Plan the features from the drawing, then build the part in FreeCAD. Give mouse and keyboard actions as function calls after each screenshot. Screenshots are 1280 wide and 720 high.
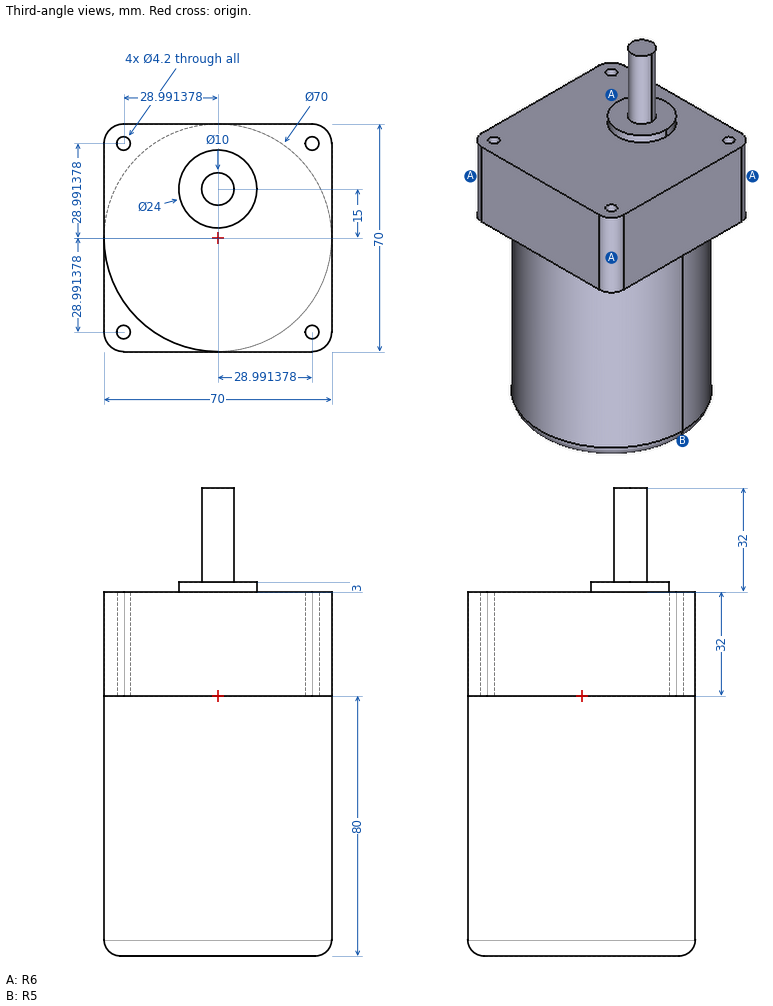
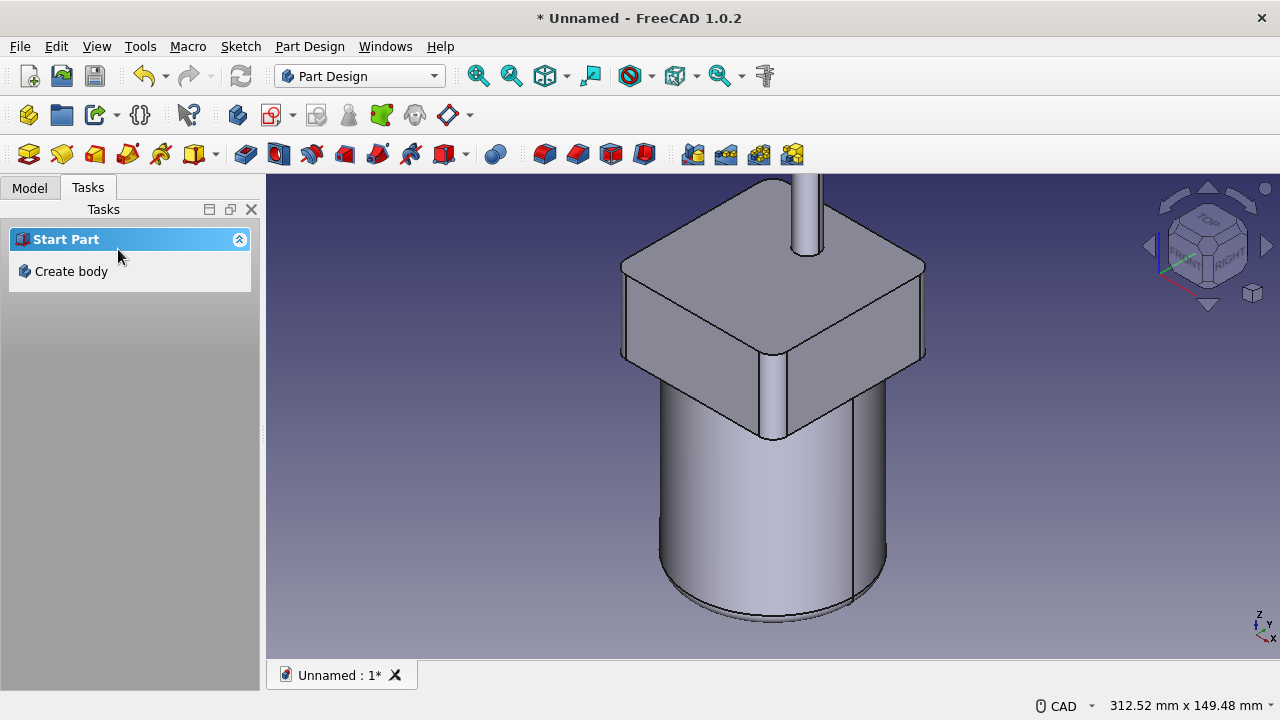
click(479, 76)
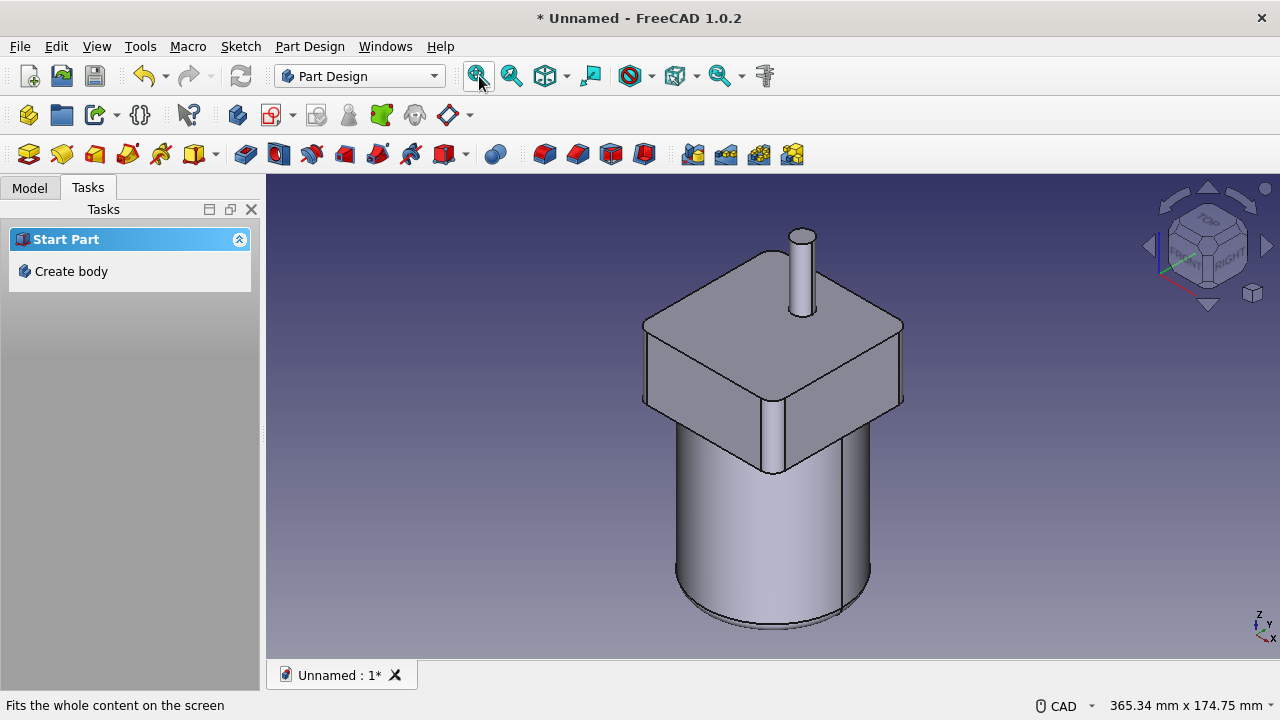
click(773, 348)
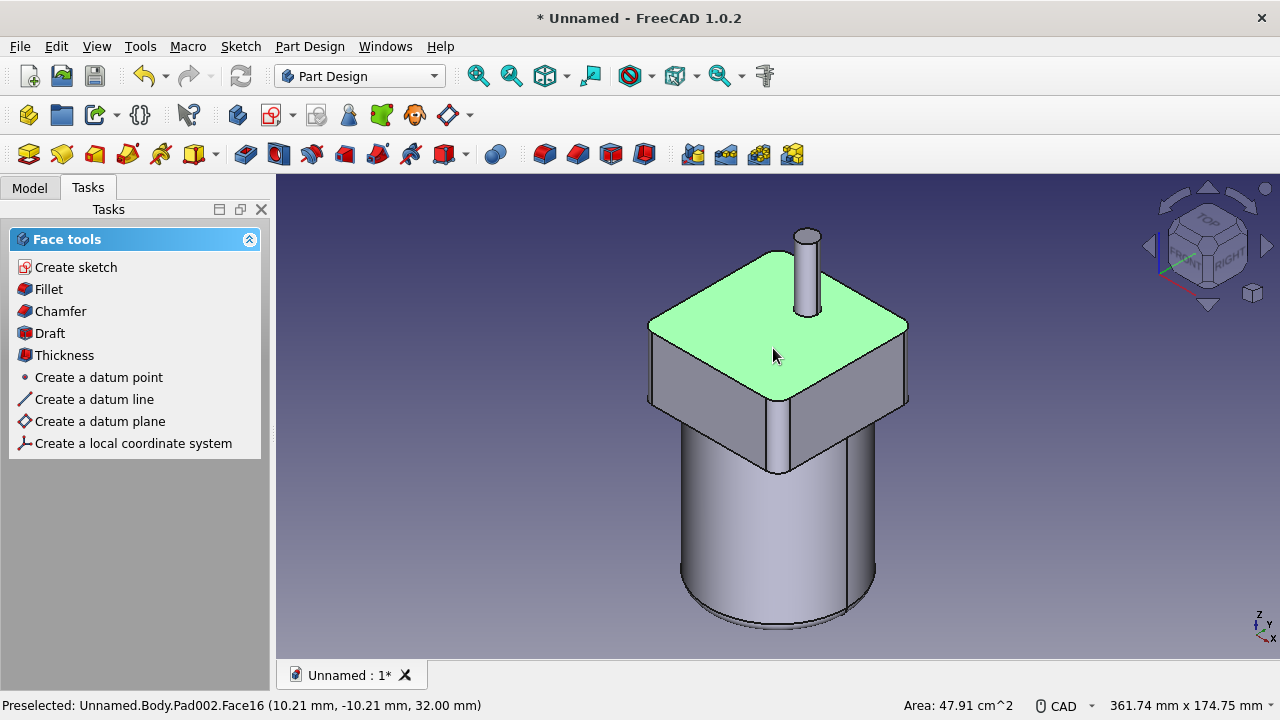
click(270, 116)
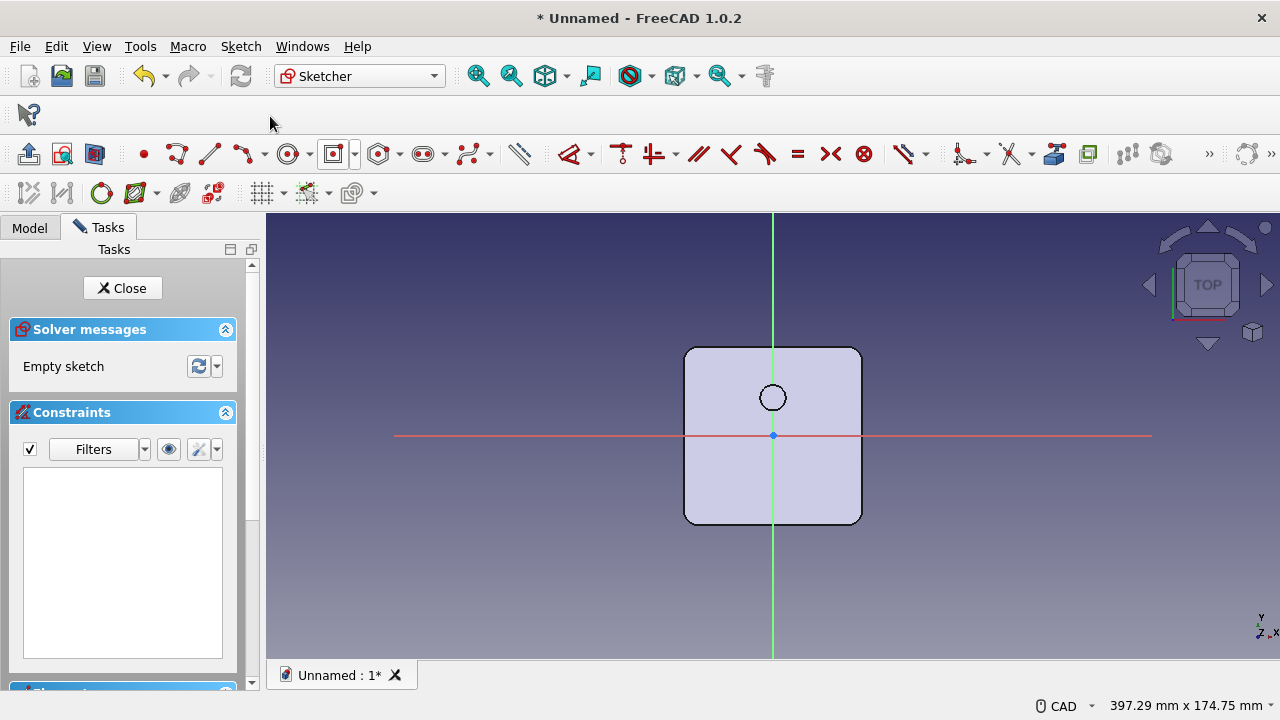
click(95, 154)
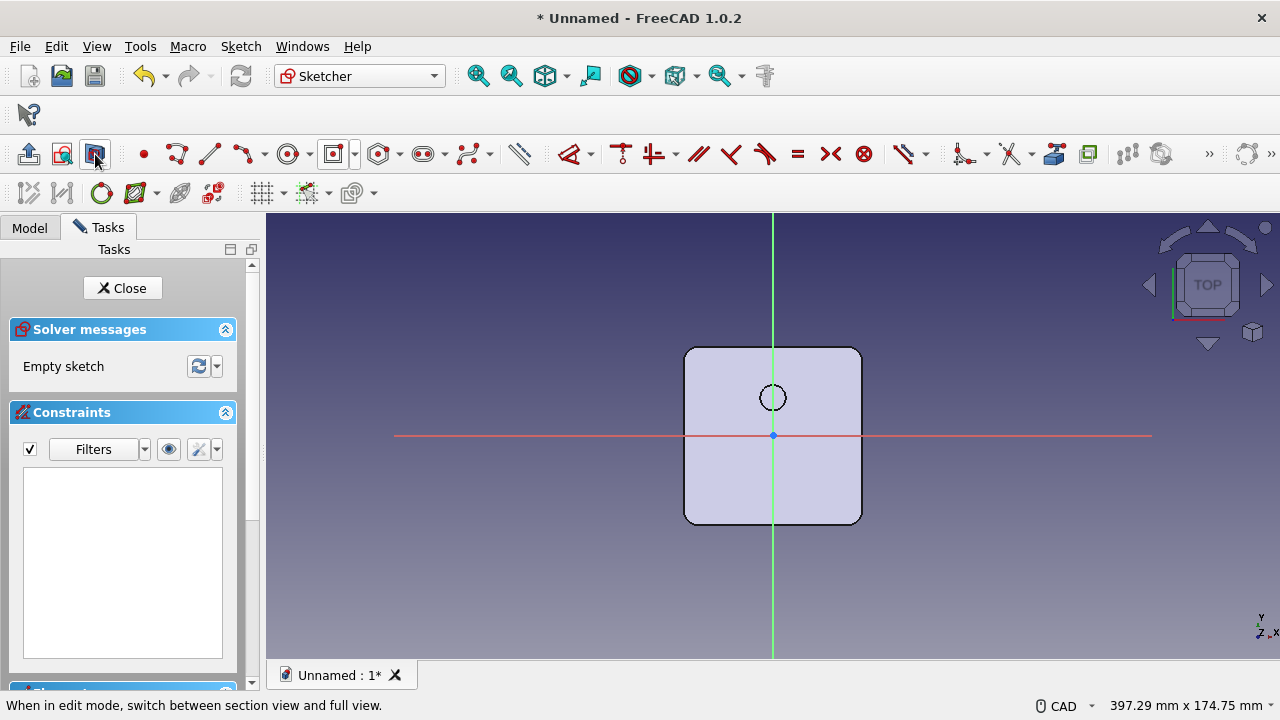
scroll(856, 436, up, 3)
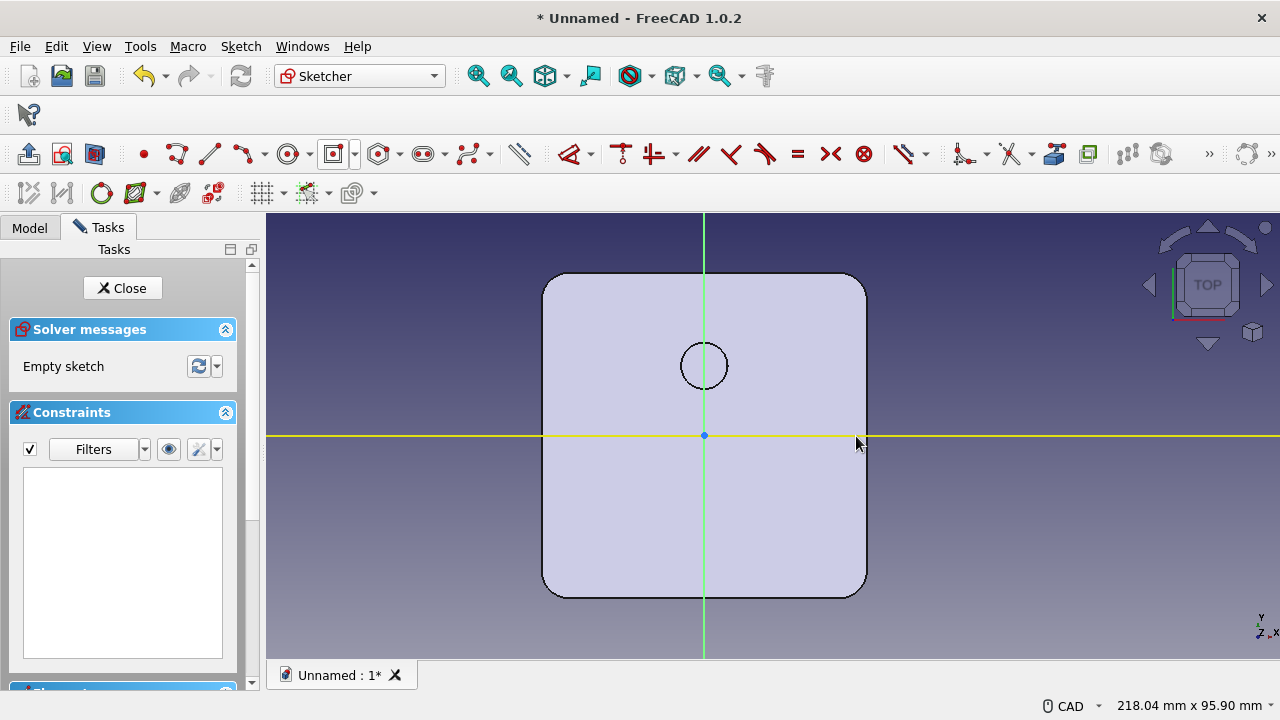
click(288, 154)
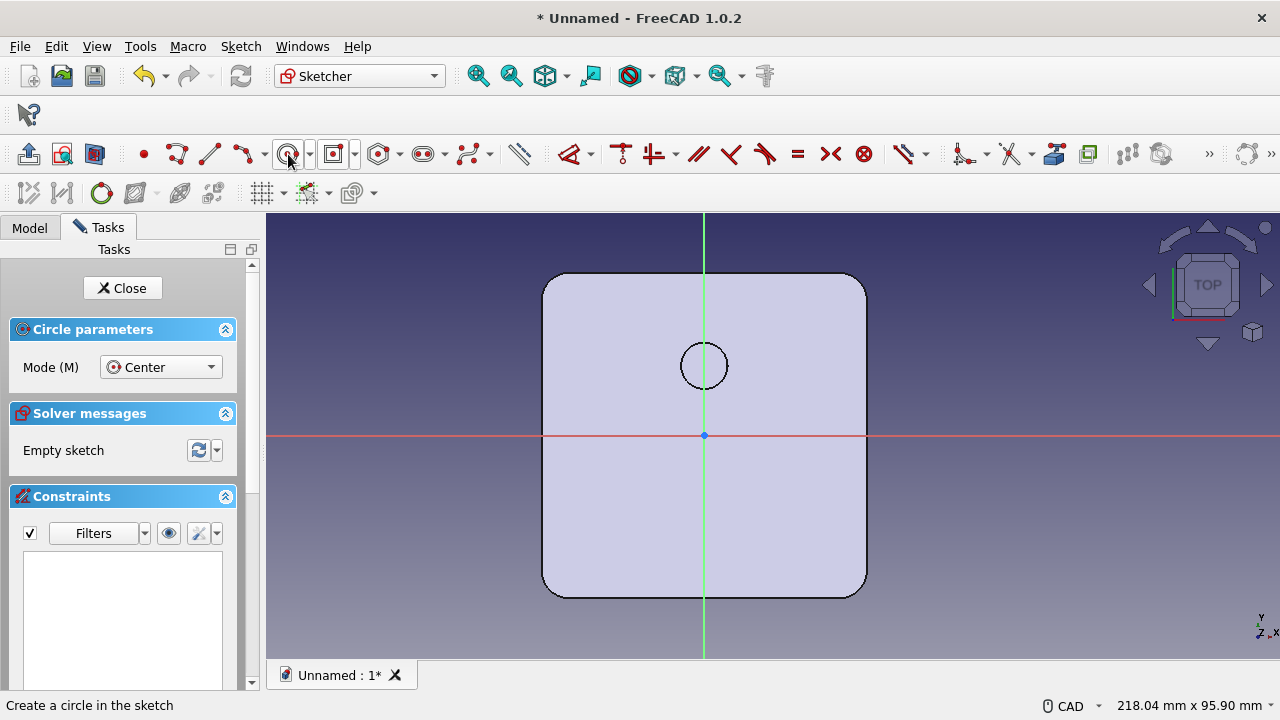
scroll(569, 301, up, 5)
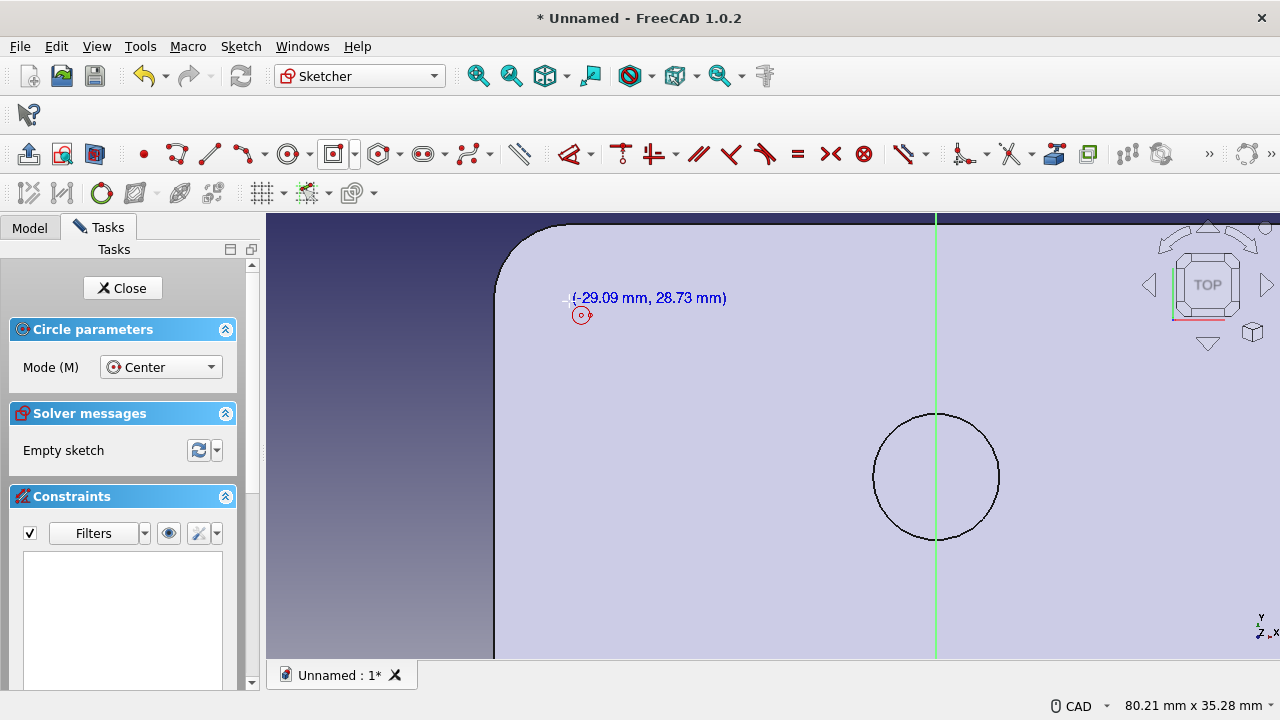
click(570, 300)
move(589, 281)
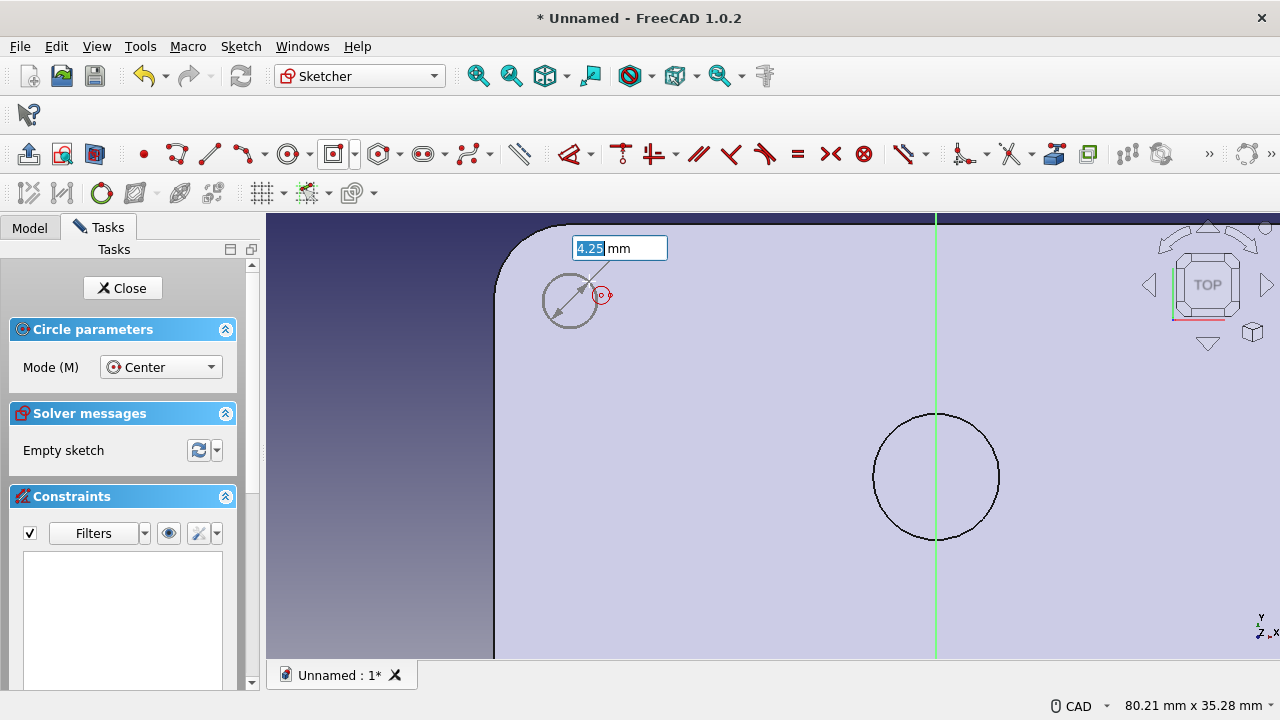
text(4.2)
key(Return)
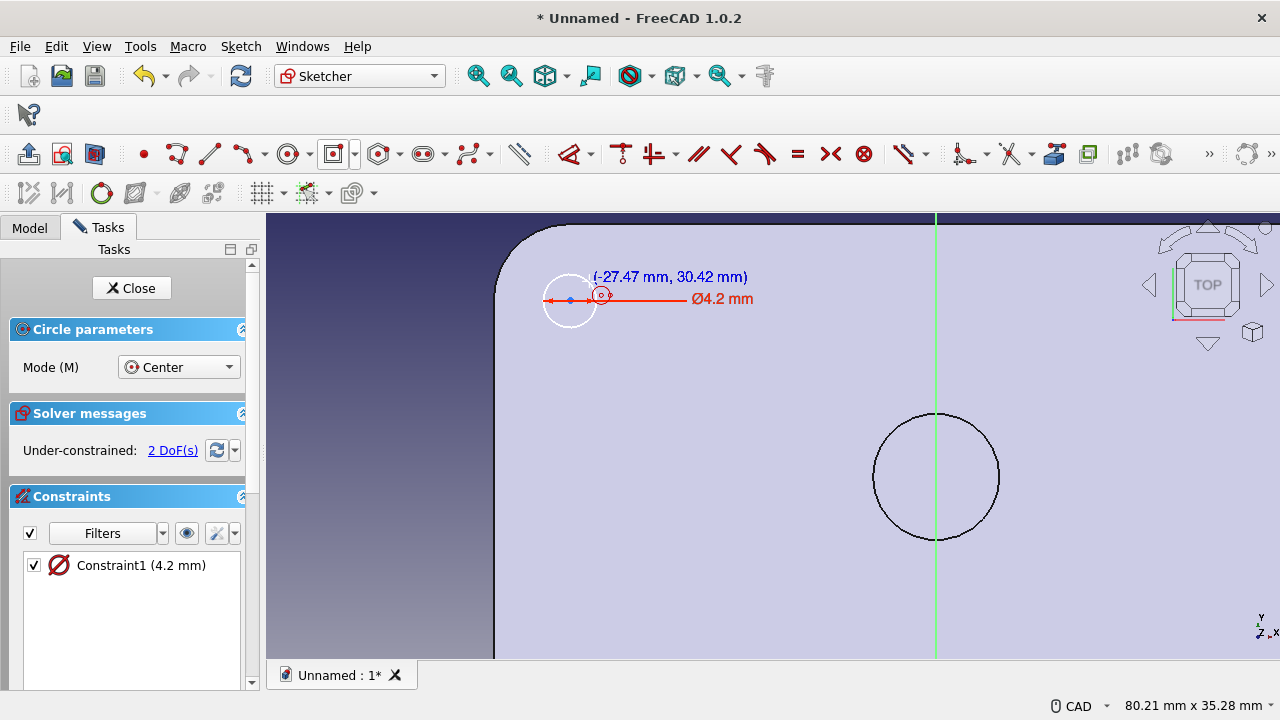
scroll(570, 302, down, 5)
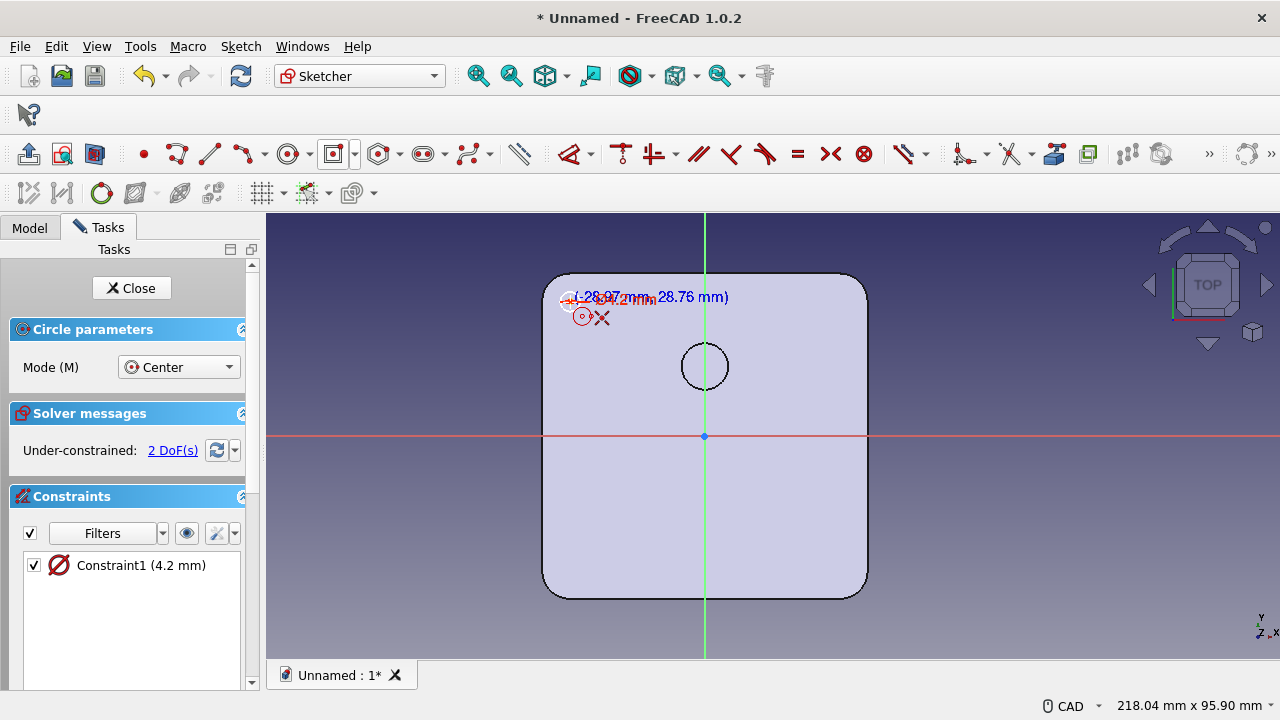
scroll(570, 571, up, 5)